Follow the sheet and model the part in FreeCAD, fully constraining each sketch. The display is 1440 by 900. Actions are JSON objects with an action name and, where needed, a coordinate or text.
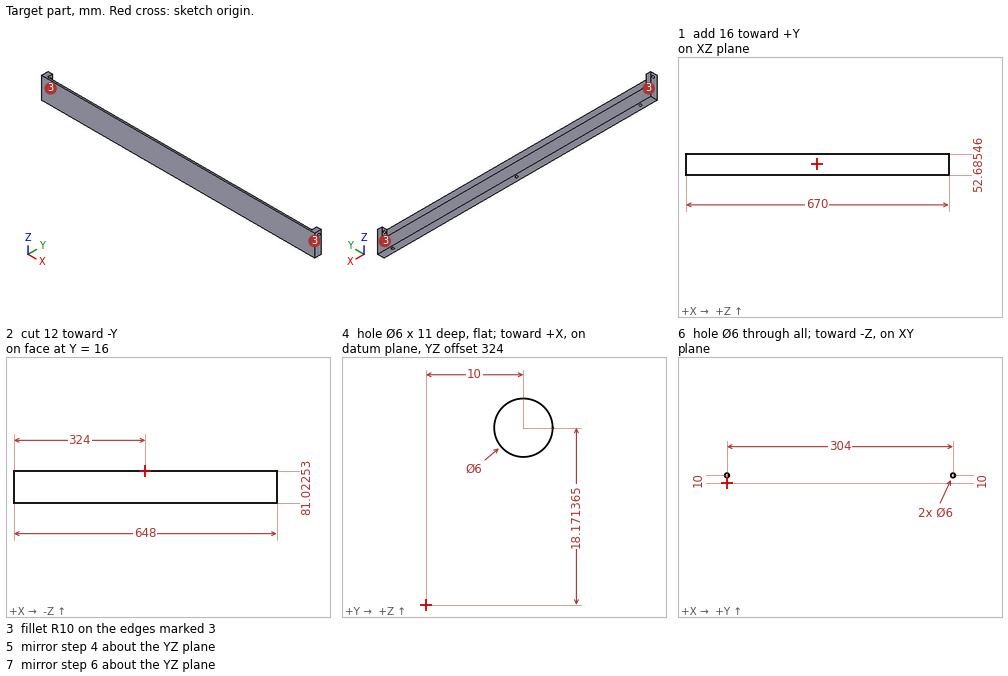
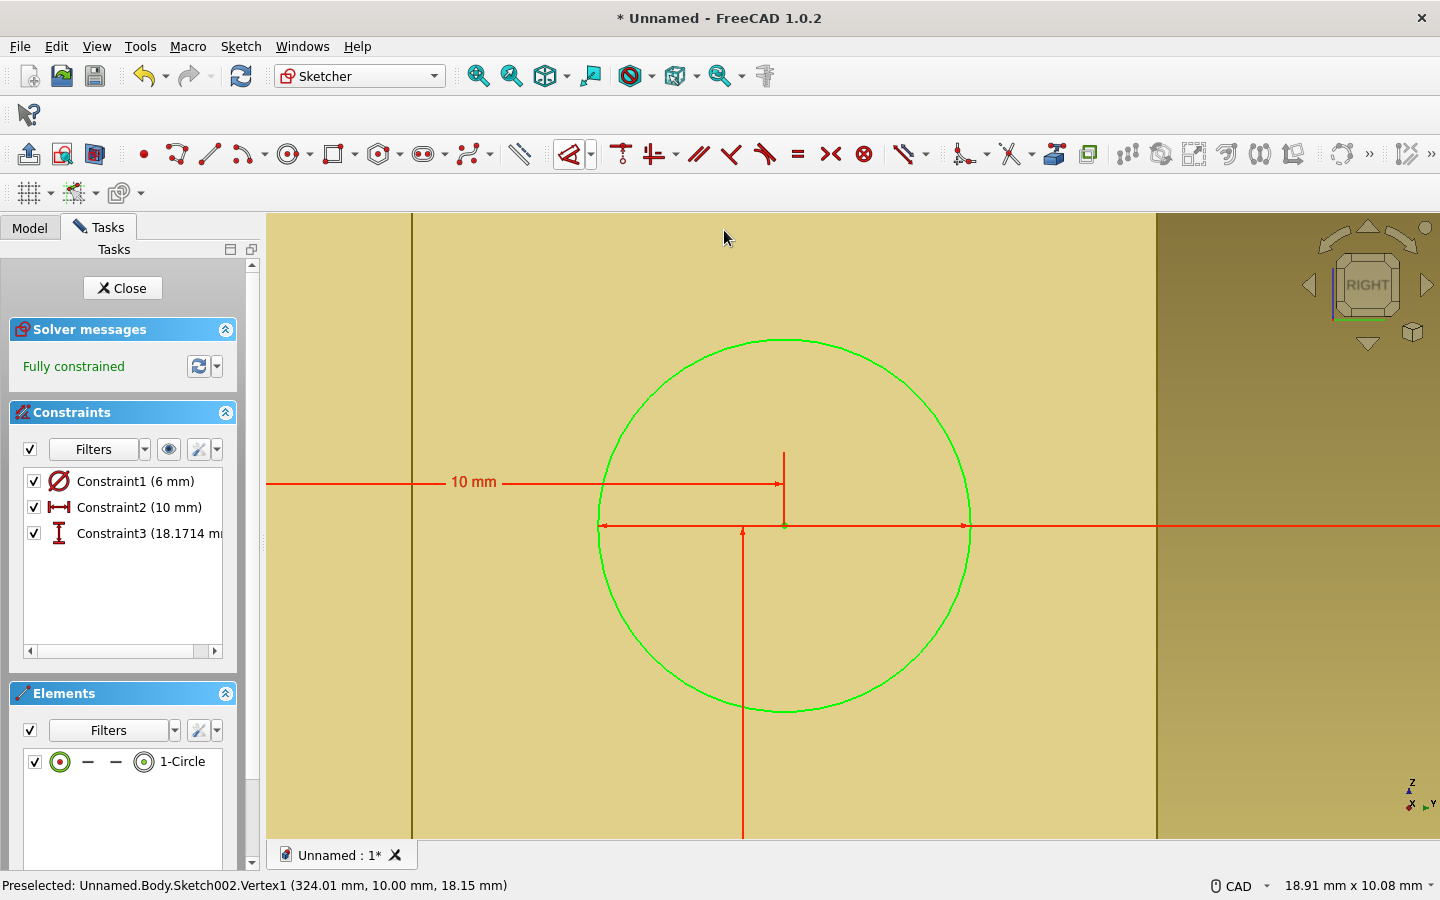
{"action": "left_click", "coordinate": [123, 288]}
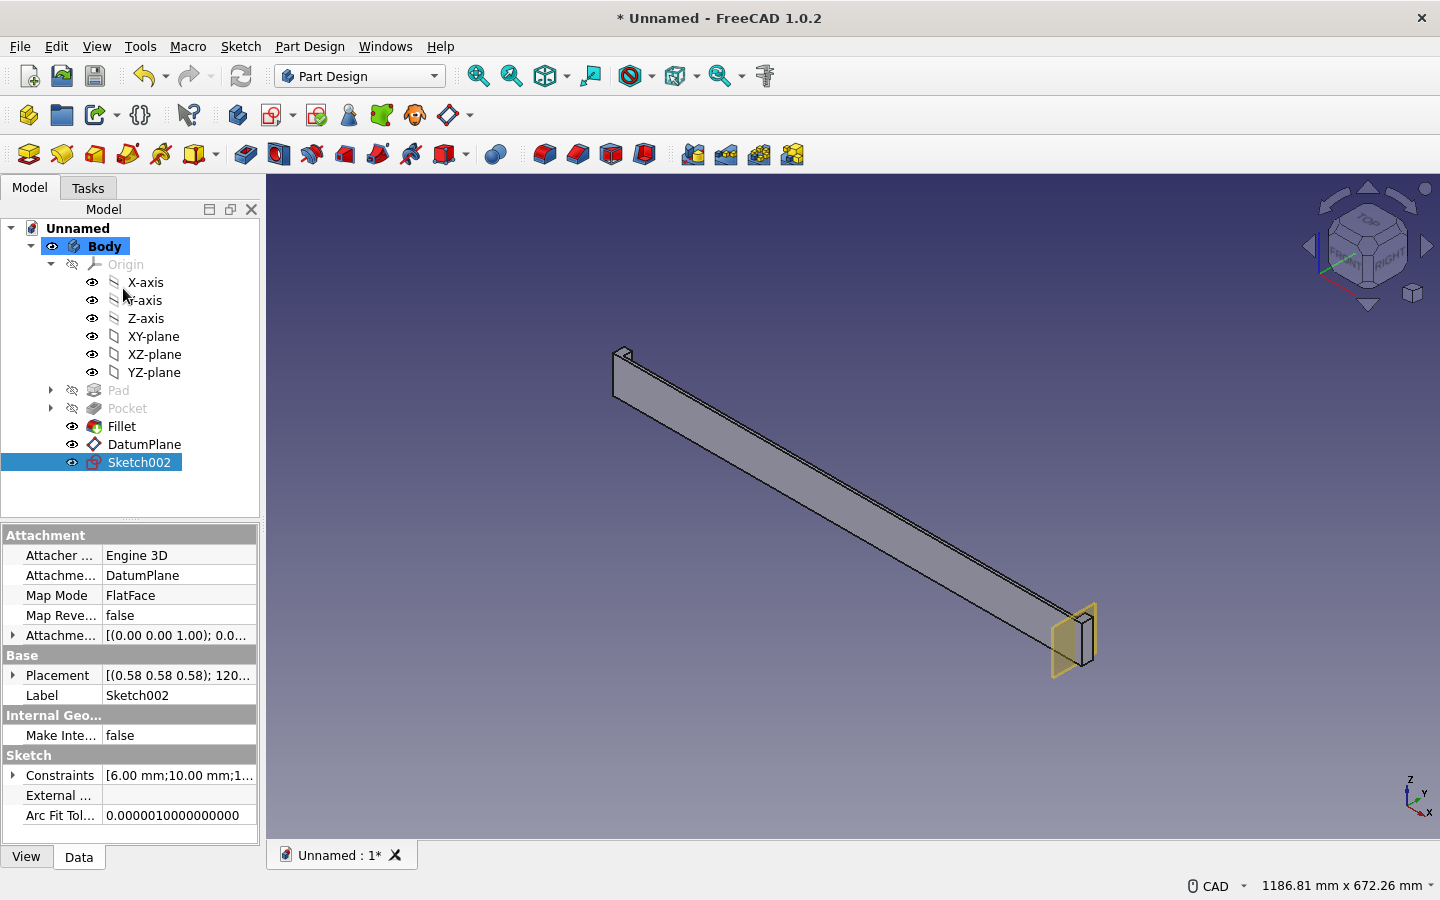
{"action": "left_click", "coordinate": [279, 154]}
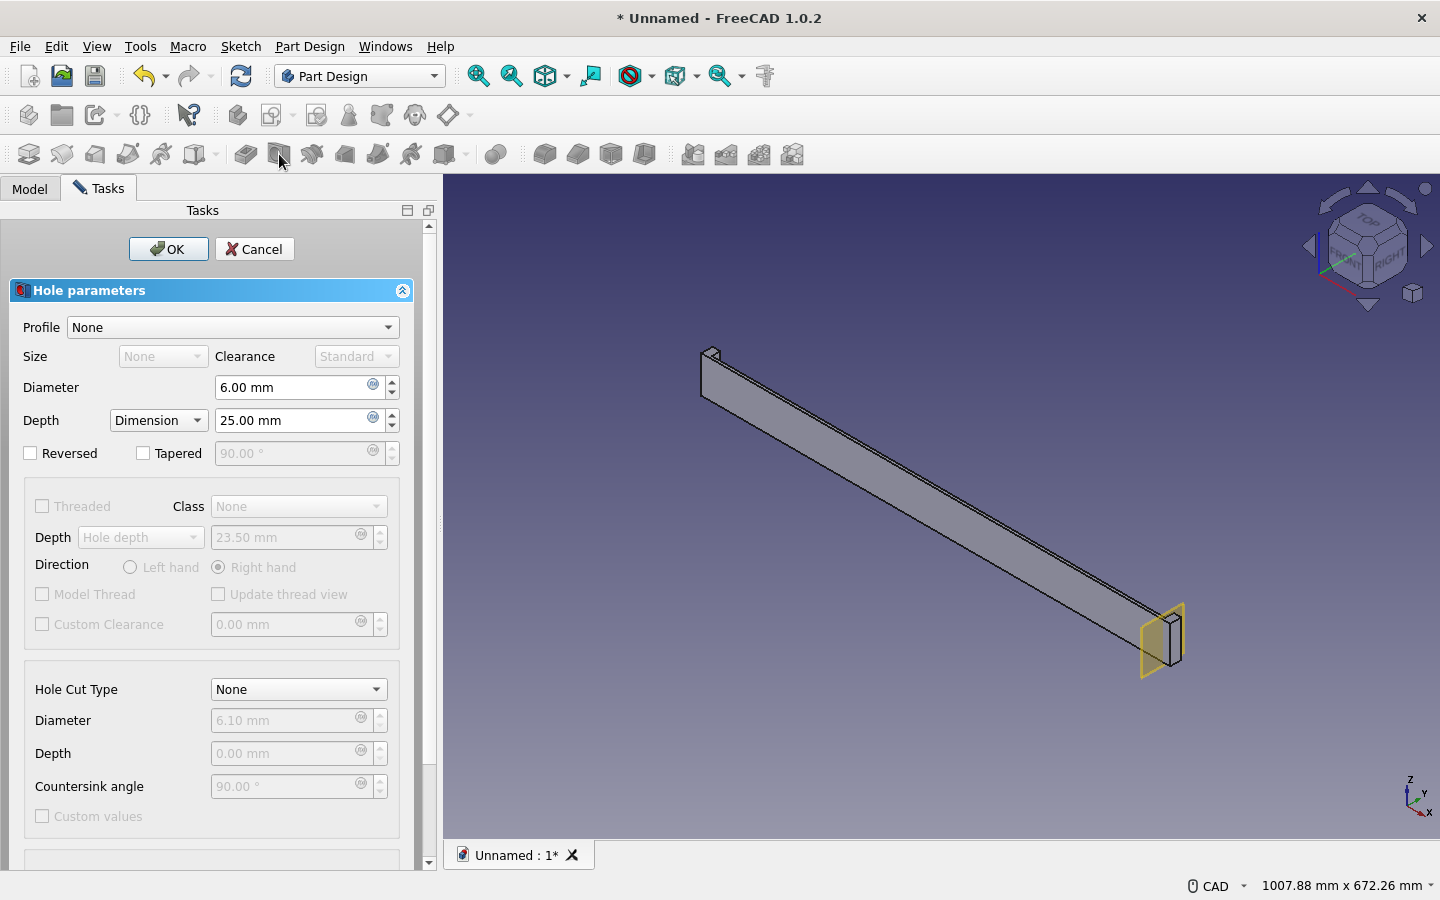
{"action": "triple_click", "coordinate": [300, 388]}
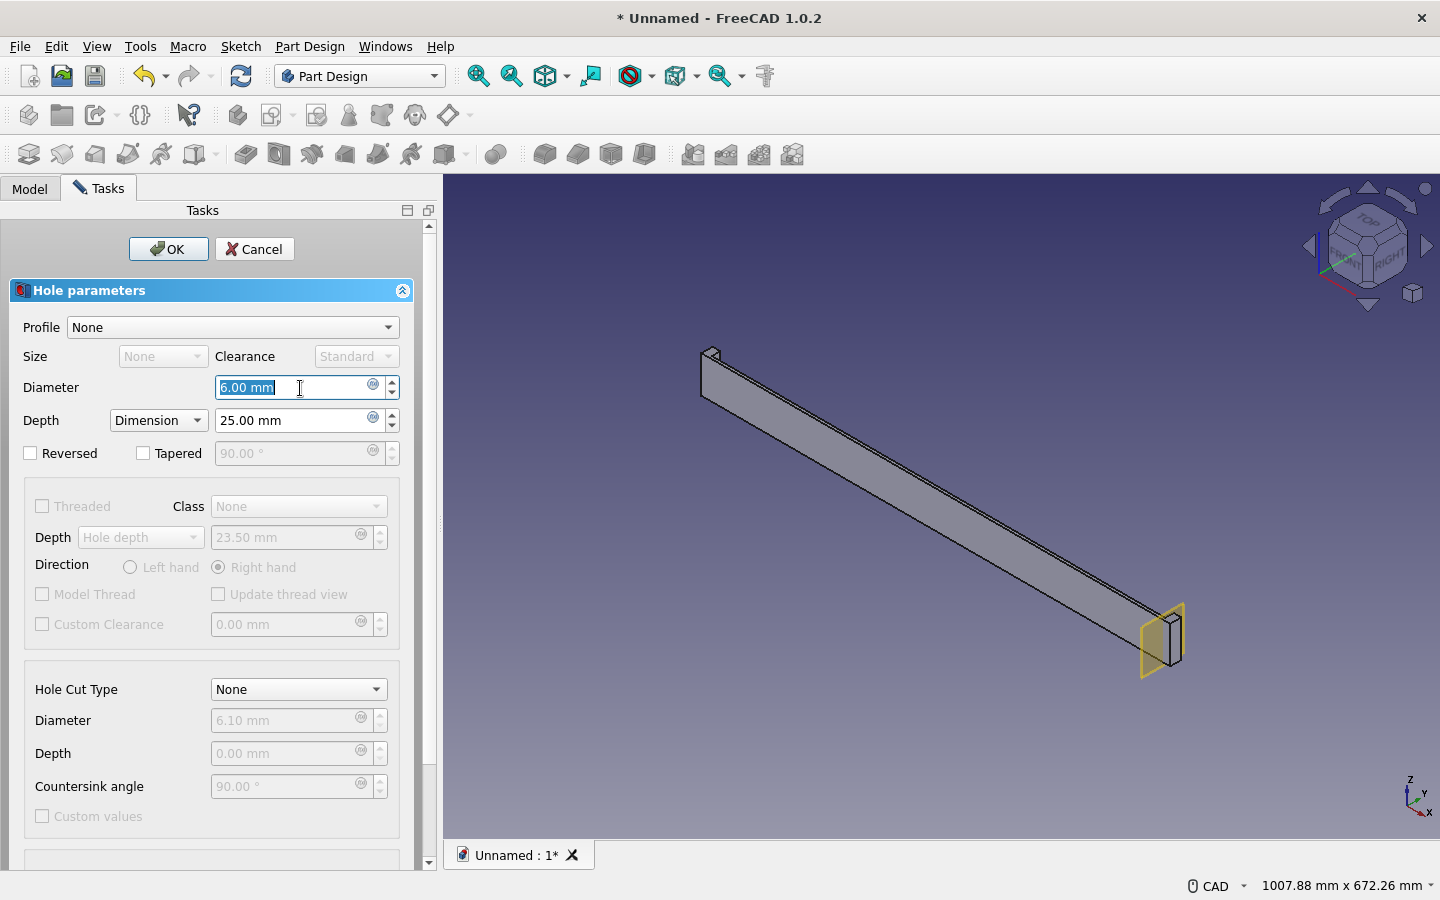
{"action": "type", "text": "6"}
{"action": "key", "text": "Tab"}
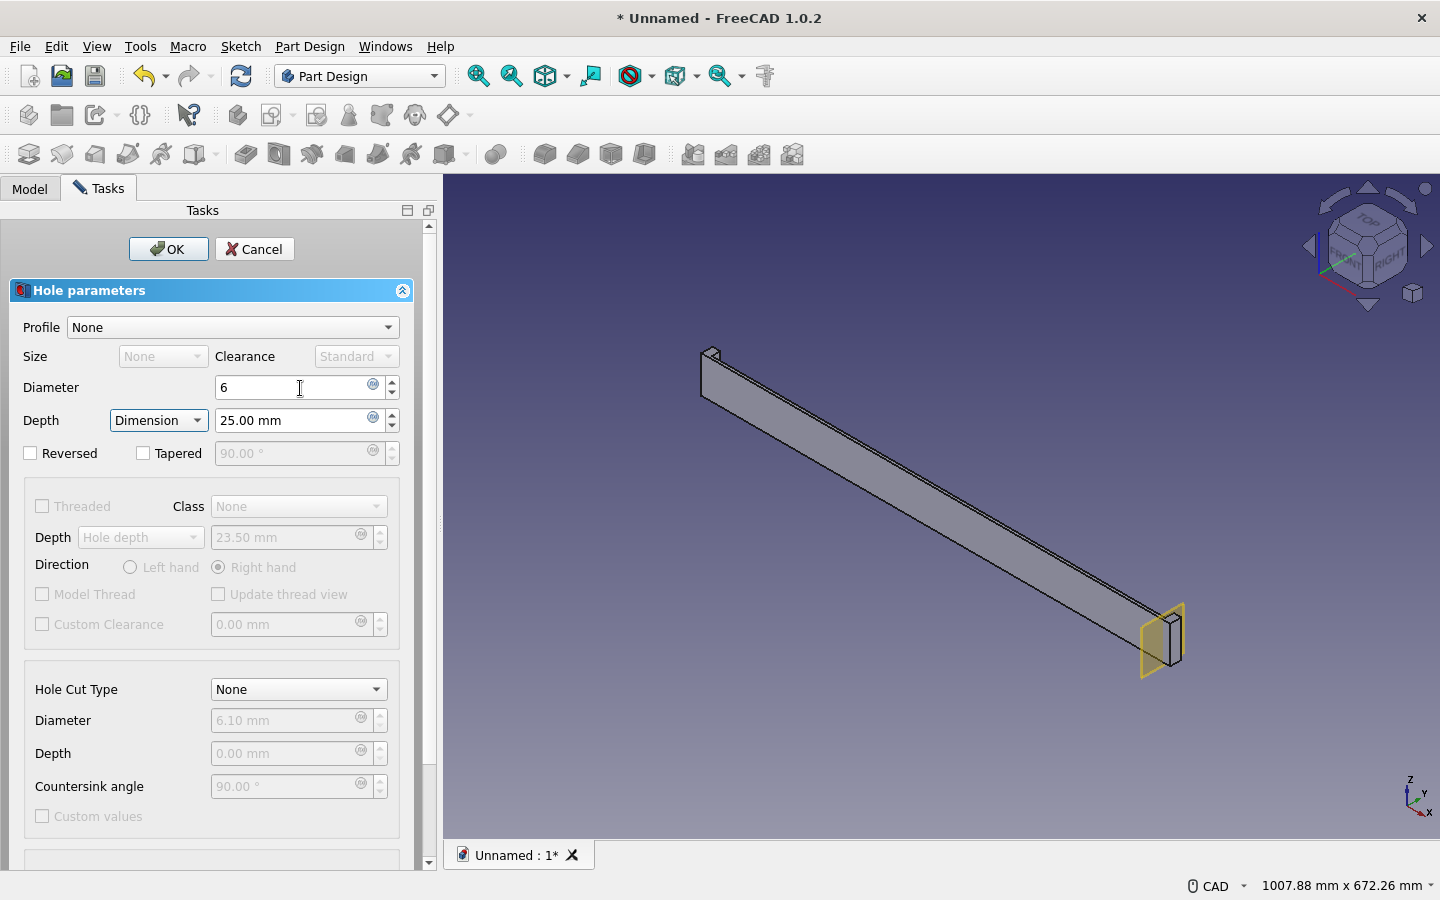
{"action": "triple_click", "coordinate": [300, 420]}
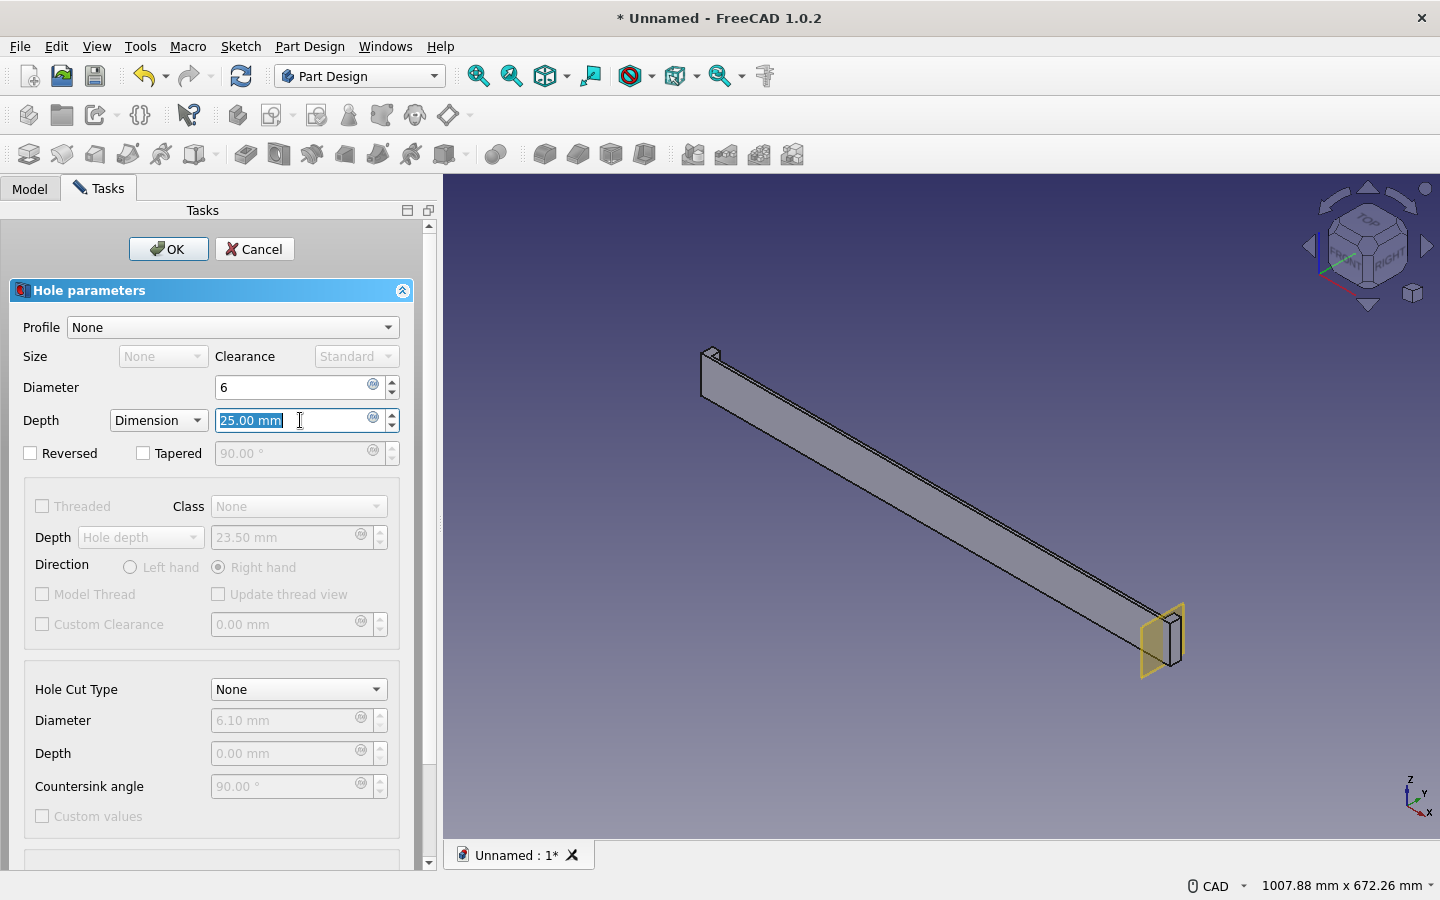
{"action": "type", "text": "11"}
{"action": "key", "text": "Tab"}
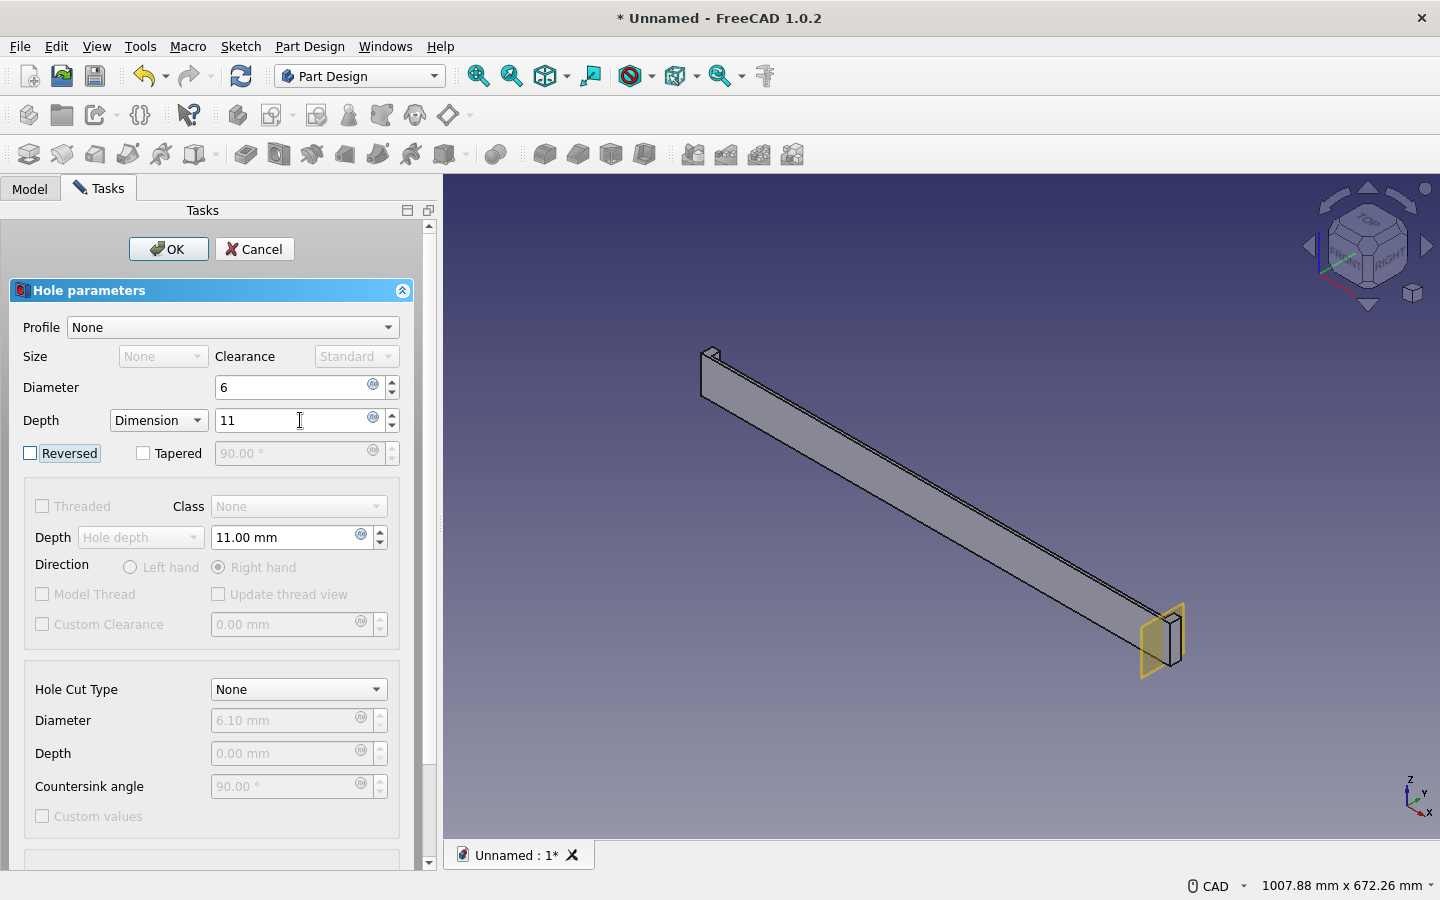
{"action": "left_click", "coordinate": [31, 453]}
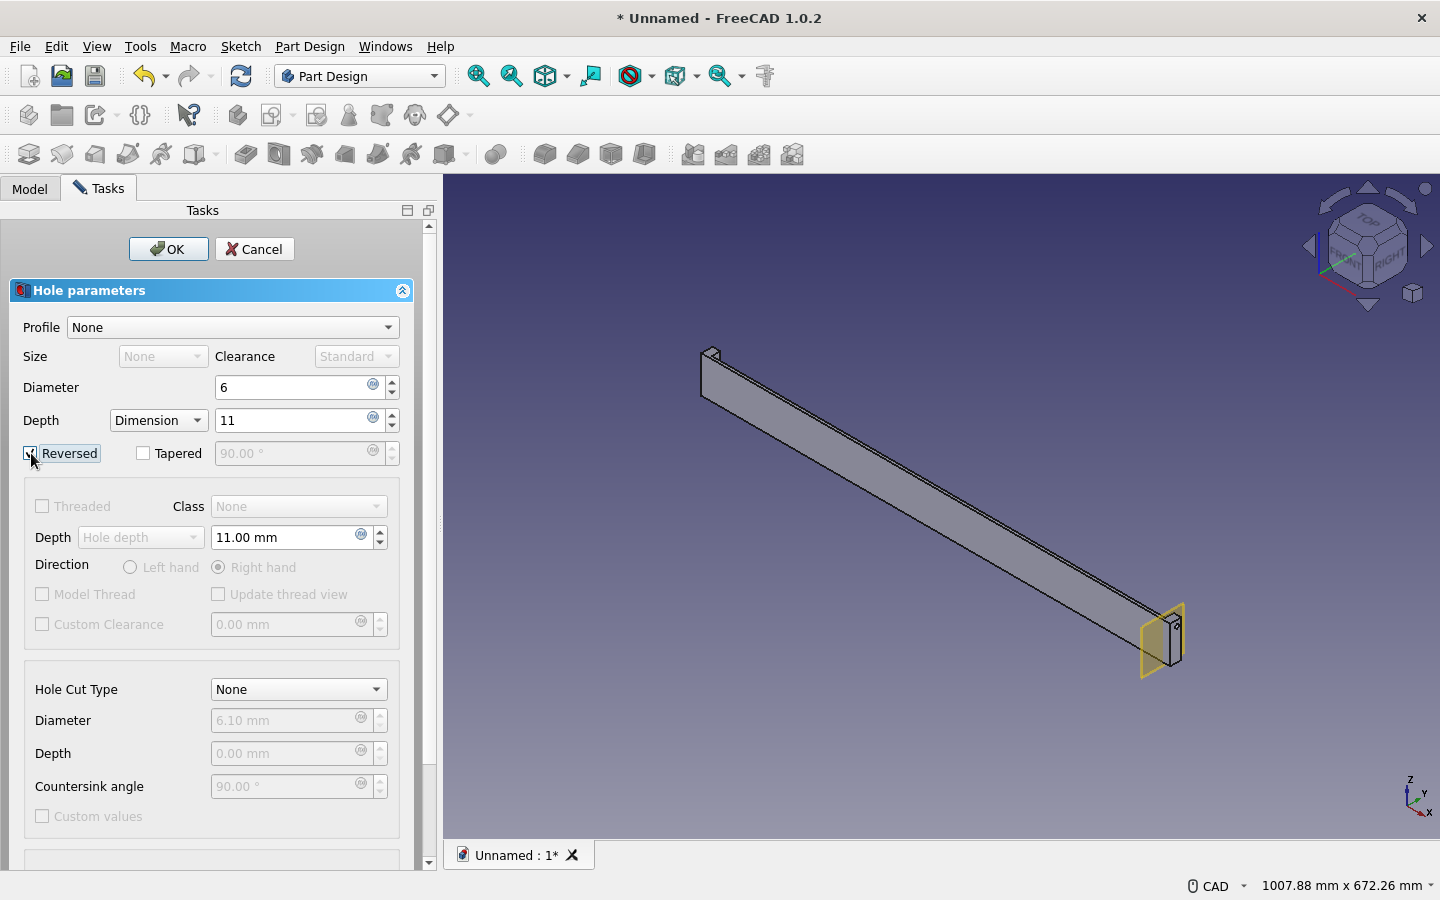
{"action": "scroll", "coordinate": [429, 545], "scroll_direction": "down", "scroll_amount": 2}